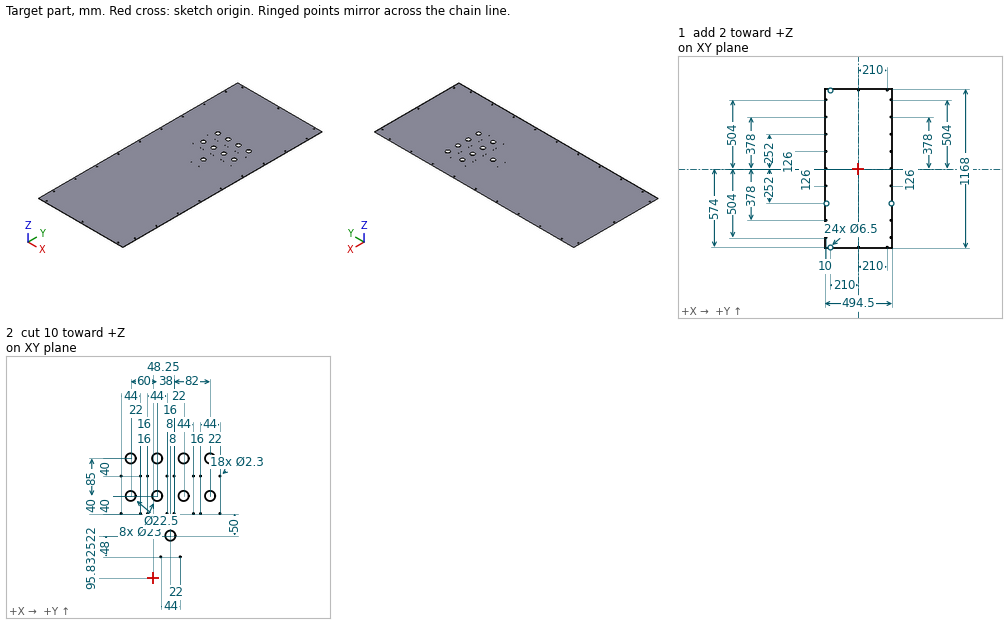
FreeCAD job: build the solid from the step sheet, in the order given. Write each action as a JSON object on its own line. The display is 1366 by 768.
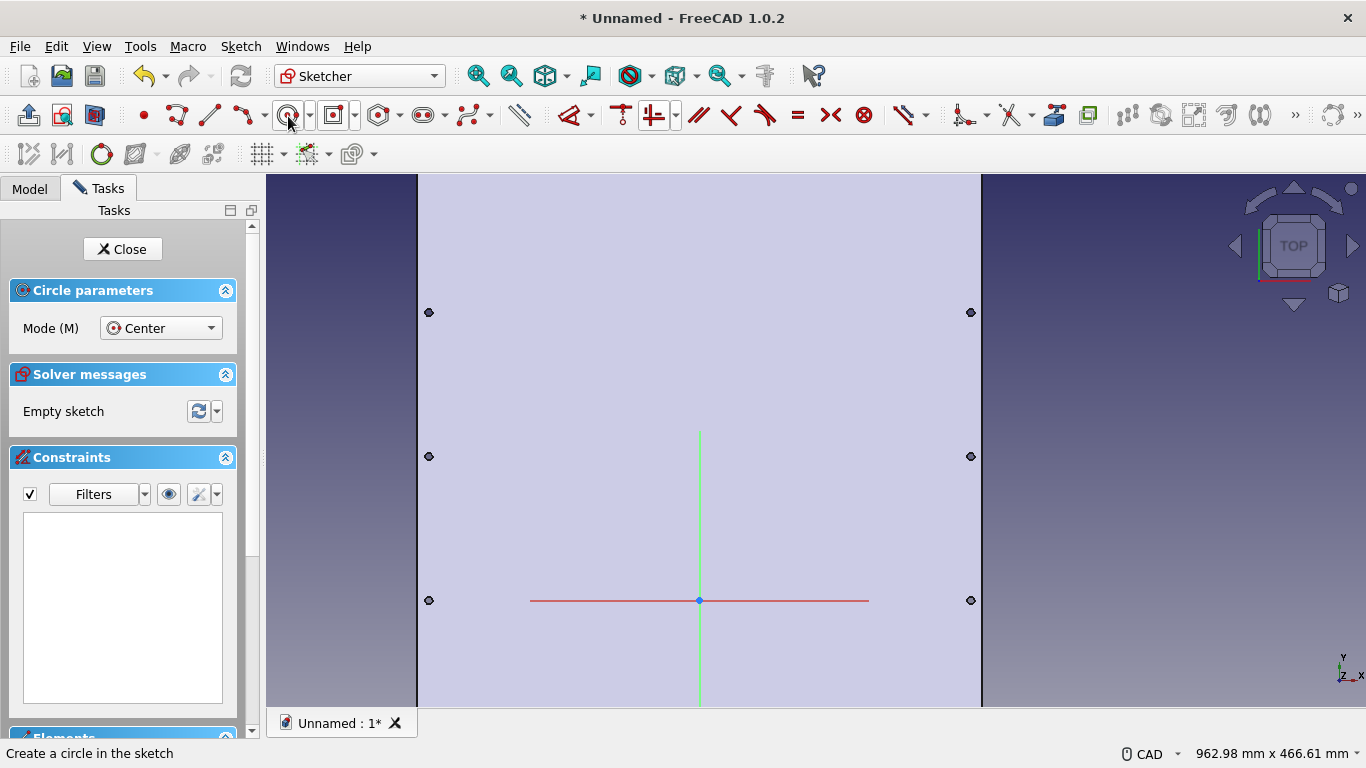
{"action": "scroll", "coordinate": [755, 434], "scroll_direction": "up", "scroll_amount": 15}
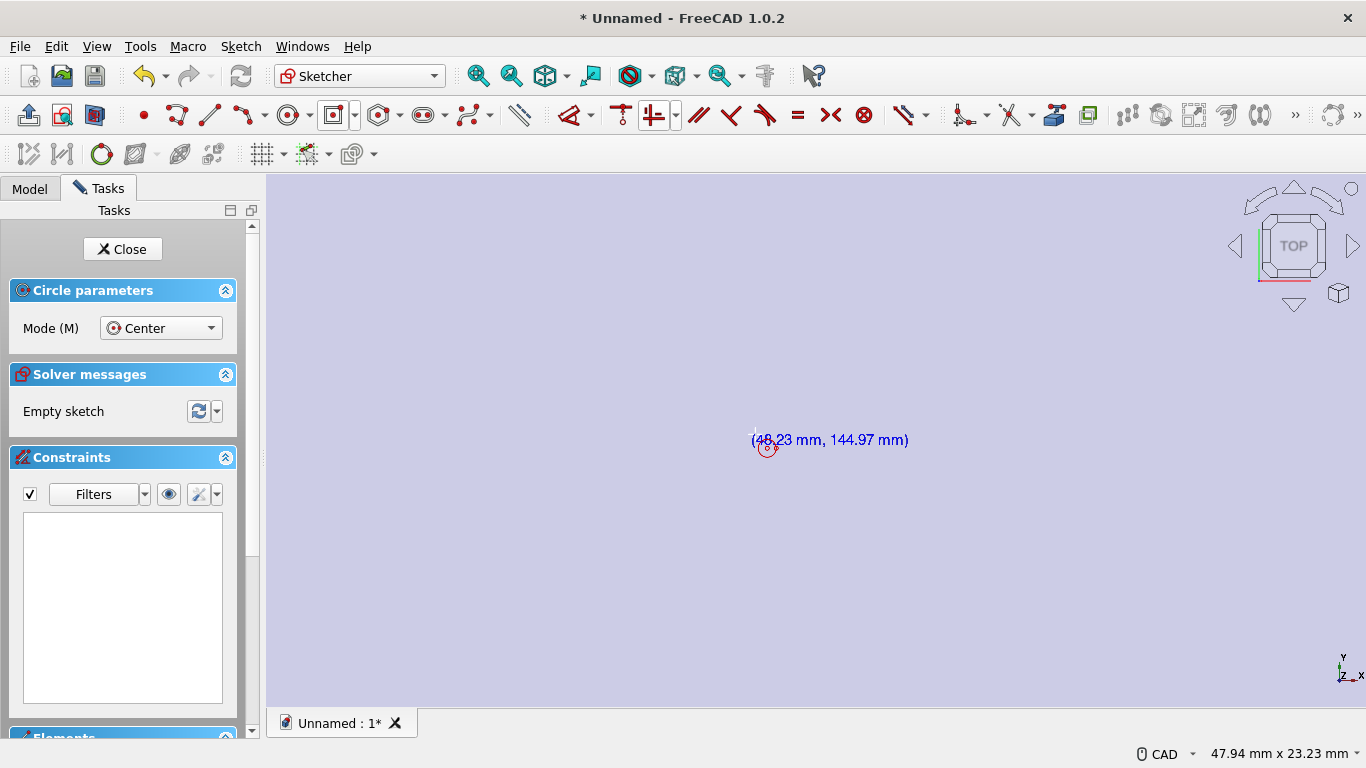
{"action": "scroll", "coordinate": [757, 436], "scroll_direction": "down", "scroll_amount": 15}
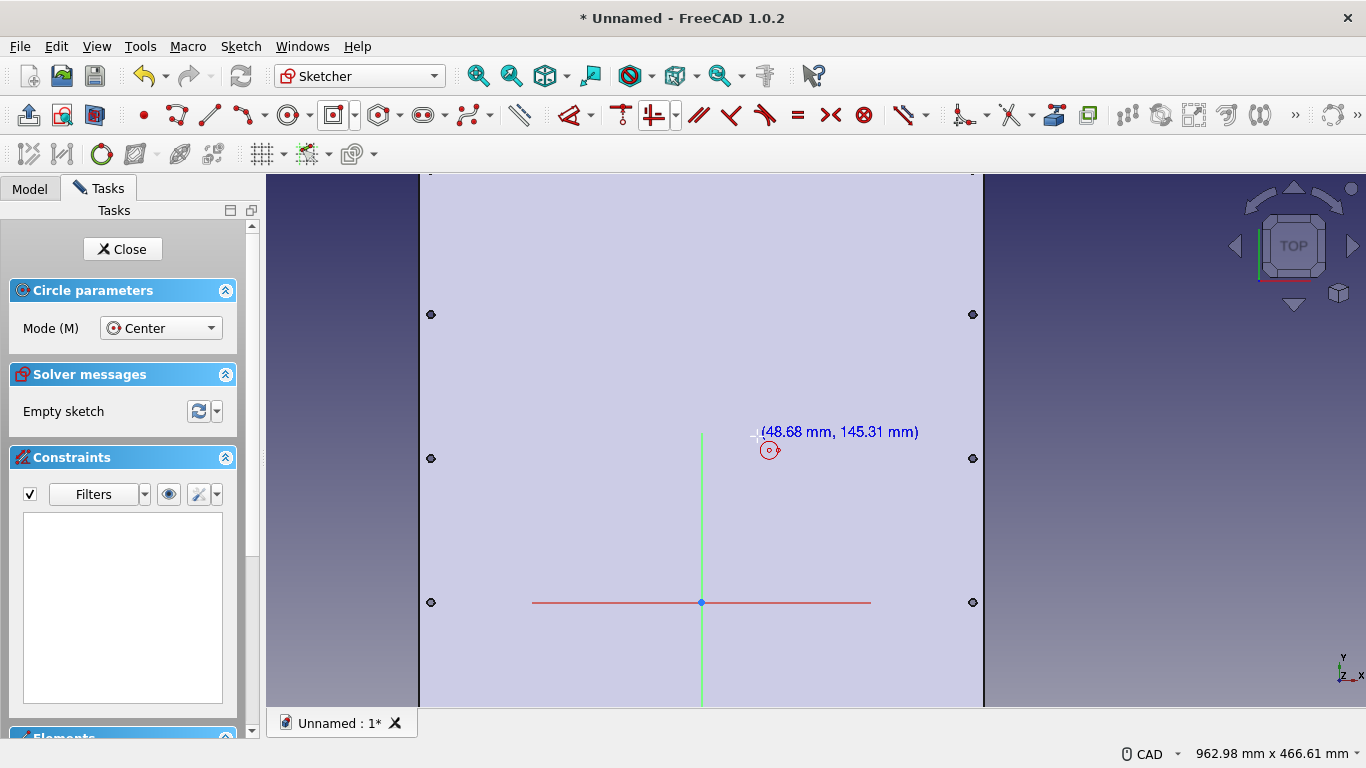
{"action": "left_click", "coordinate": [757, 436]}
{"action": "mouse_move", "coordinate": [758, 435]}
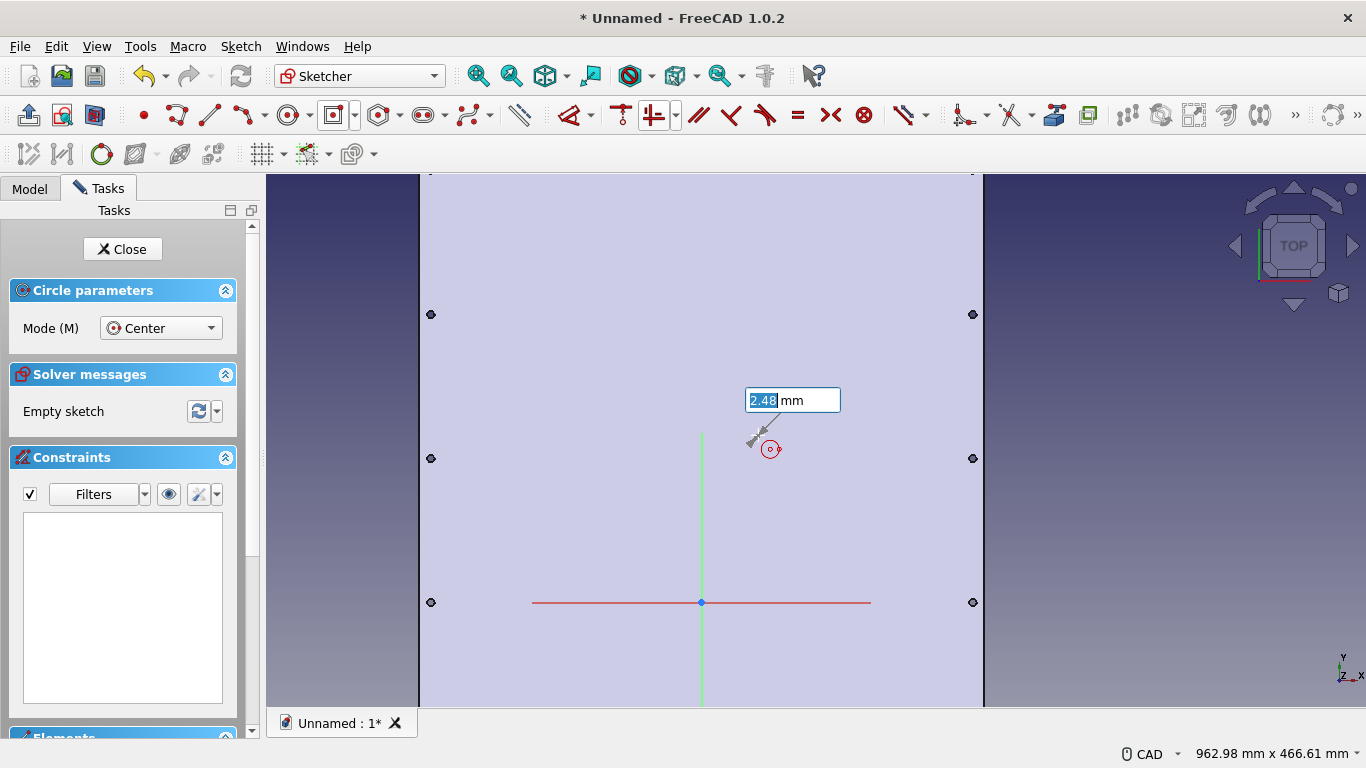
{"action": "type", "text": "2.3"}
{"action": "key", "text": "Return"}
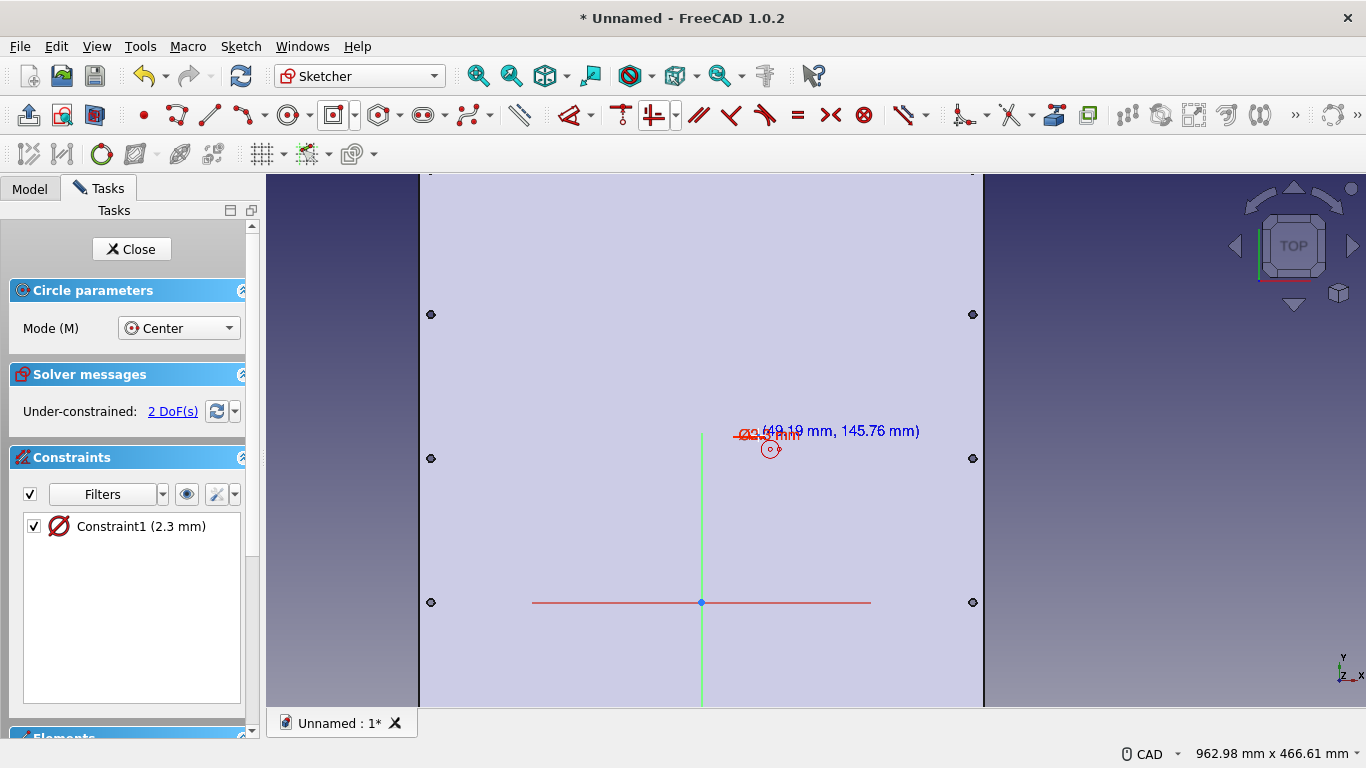
{"action": "scroll", "coordinate": [714, 390], "scroll_direction": "up", "scroll_amount": 3}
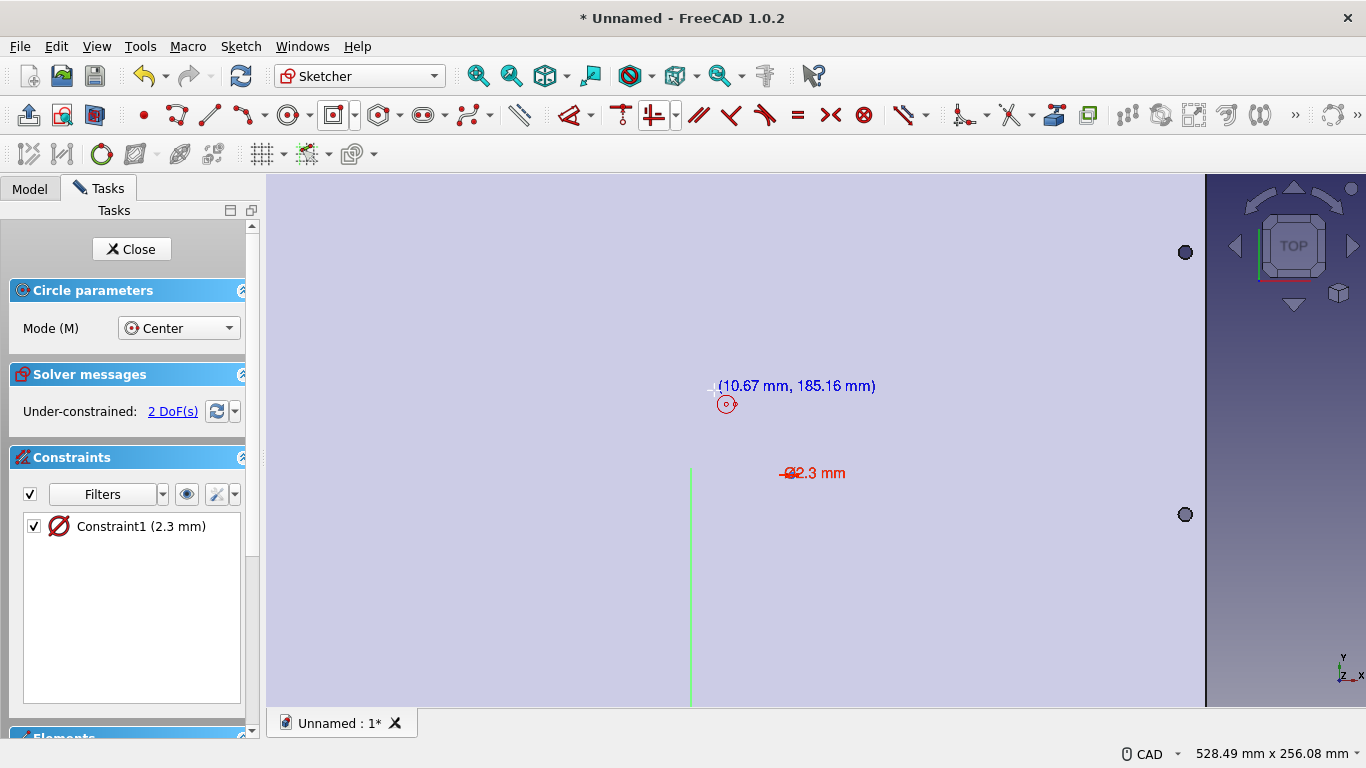
{"action": "left_click", "coordinate": [713, 390]}
{"action": "mouse_move", "coordinate": [730, 373]}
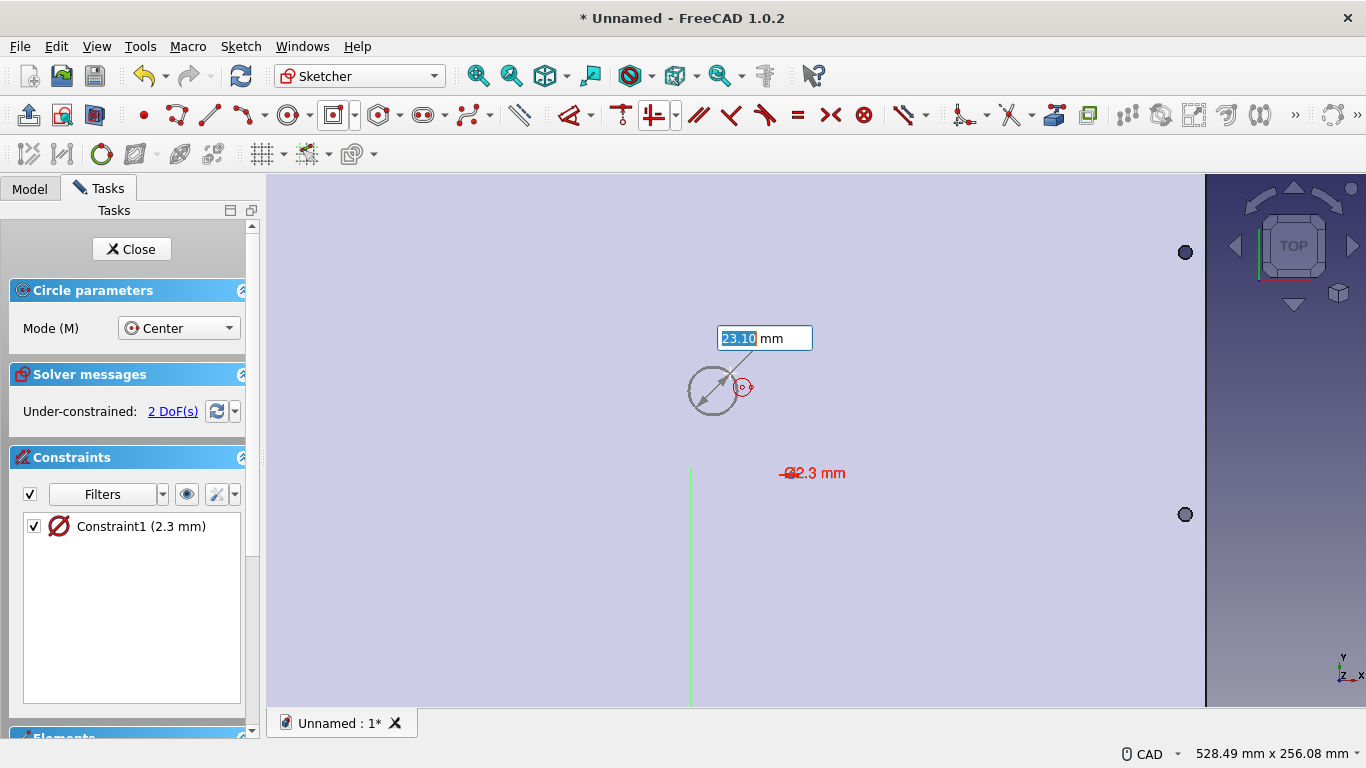
{"action": "type", "text": "23"}
{"action": "key", "text": "Return"}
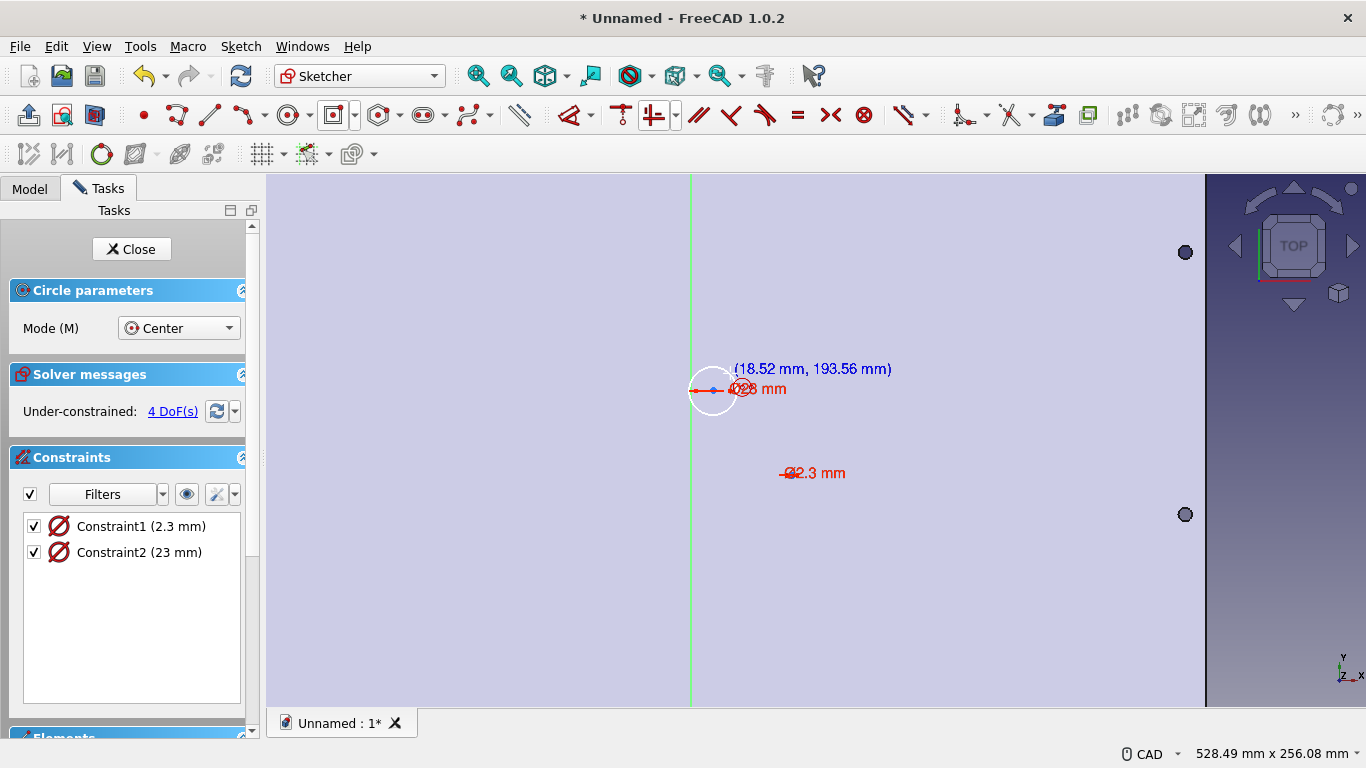
{"action": "scroll", "coordinate": [759, 473], "scroll_direction": "up", "scroll_amount": 12}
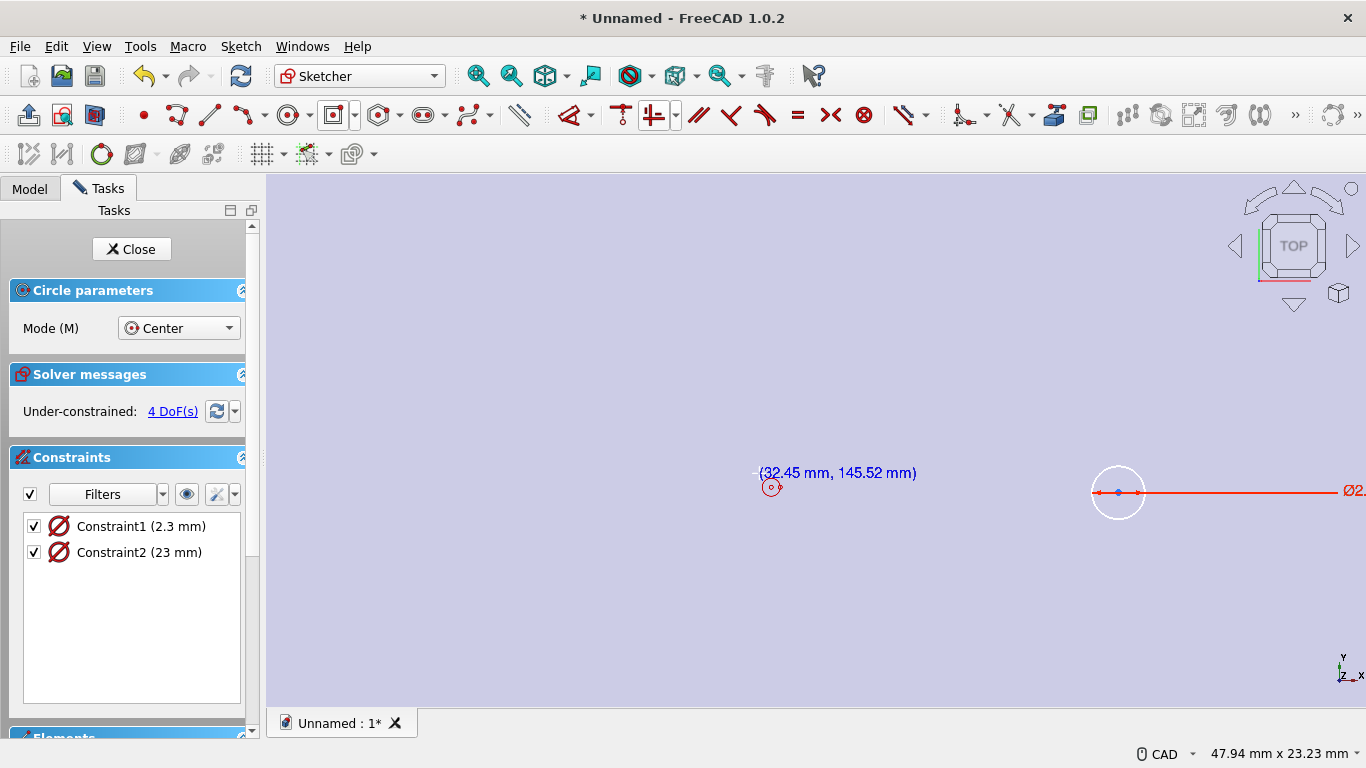
{"action": "scroll", "coordinate": [738, 433], "scroll_direction": "down", "scroll_amount": 15}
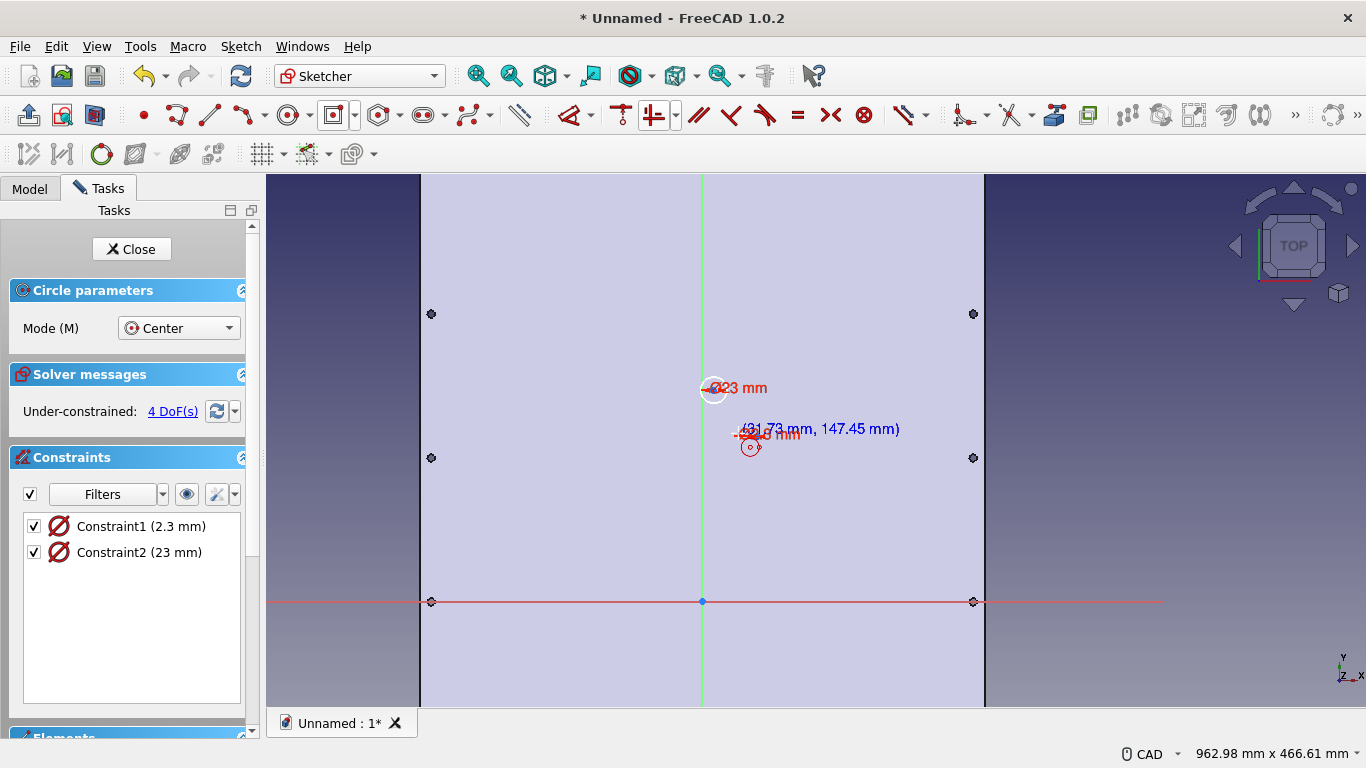
{"action": "left_click", "coordinate": [739, 435]}
{"action": "mouse_move", "coordinate": [740, 434]}